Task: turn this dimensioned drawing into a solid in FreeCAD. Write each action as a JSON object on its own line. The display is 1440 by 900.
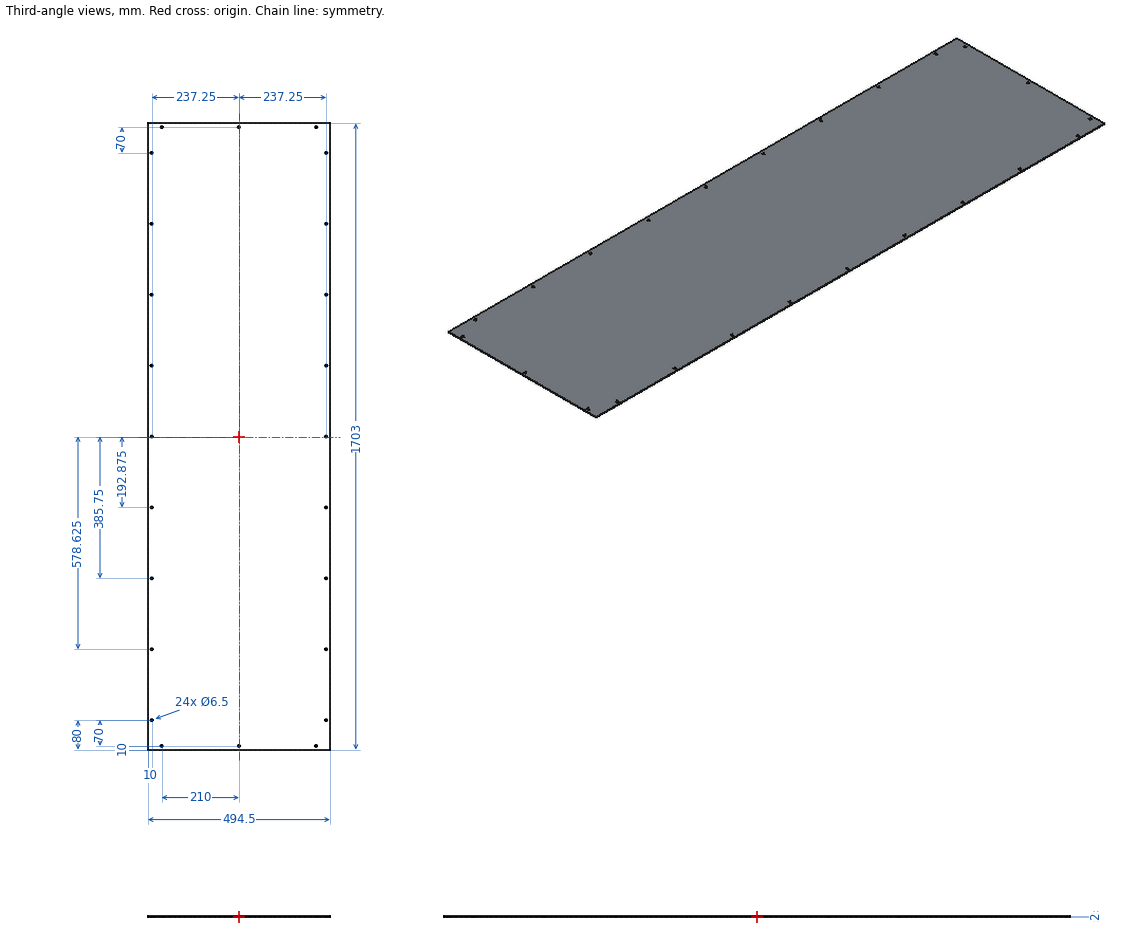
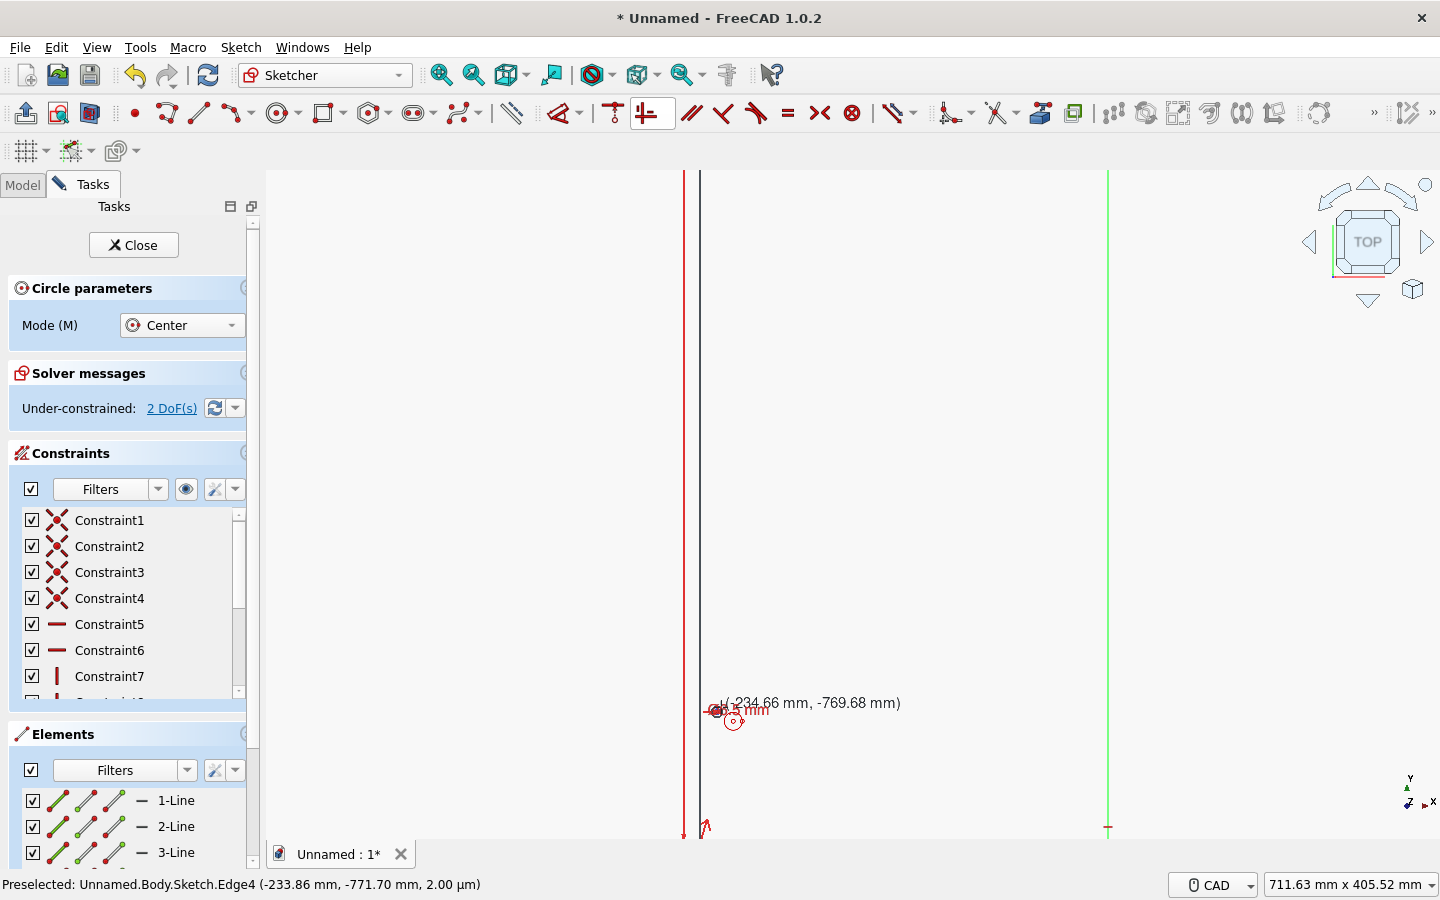
{"action": "scroll", "coordinate": [720, 716], "scroll_direction": "down", "scroll_amount": 9}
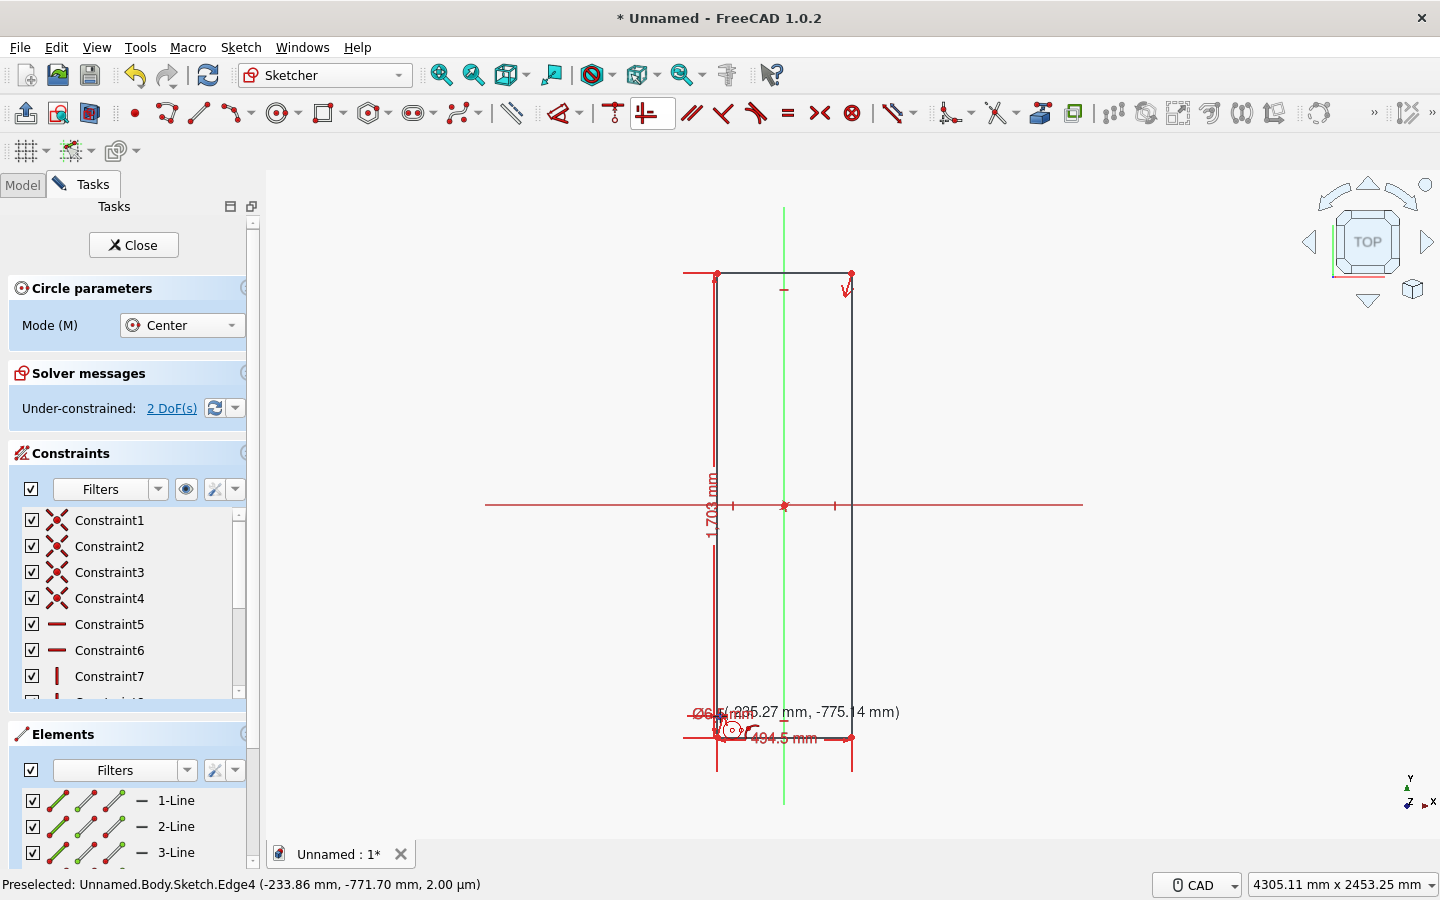
{"action": "scroll", "coordinate": [727, 735], "scroll_direction": "up", "scroll_amount": 17}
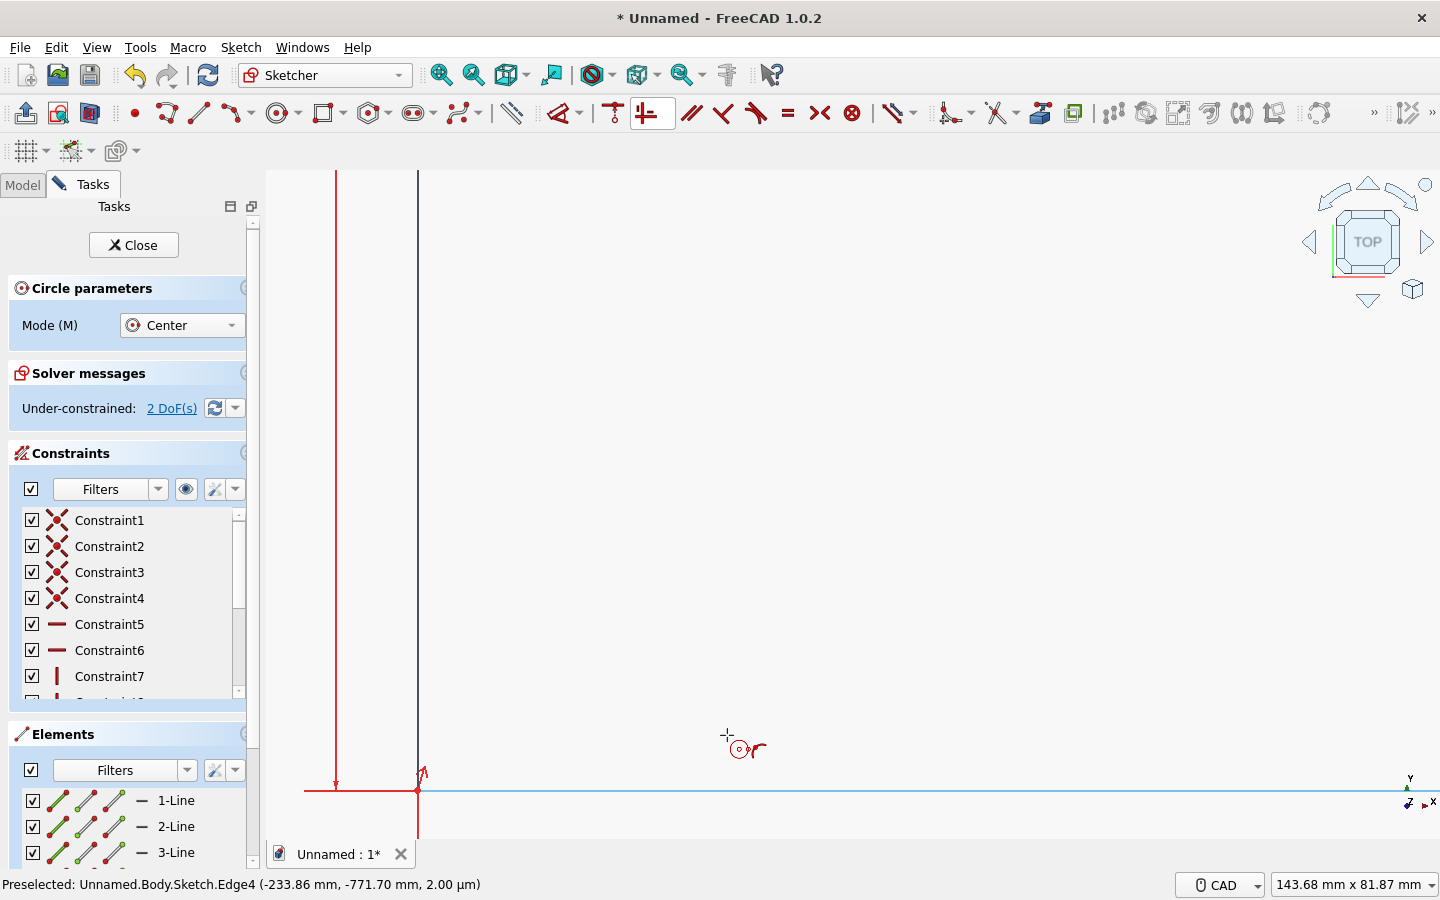
{"action": "scroll", "coordinate": [727, 735], "scroll_direction": "down", "scroll_amount": 17}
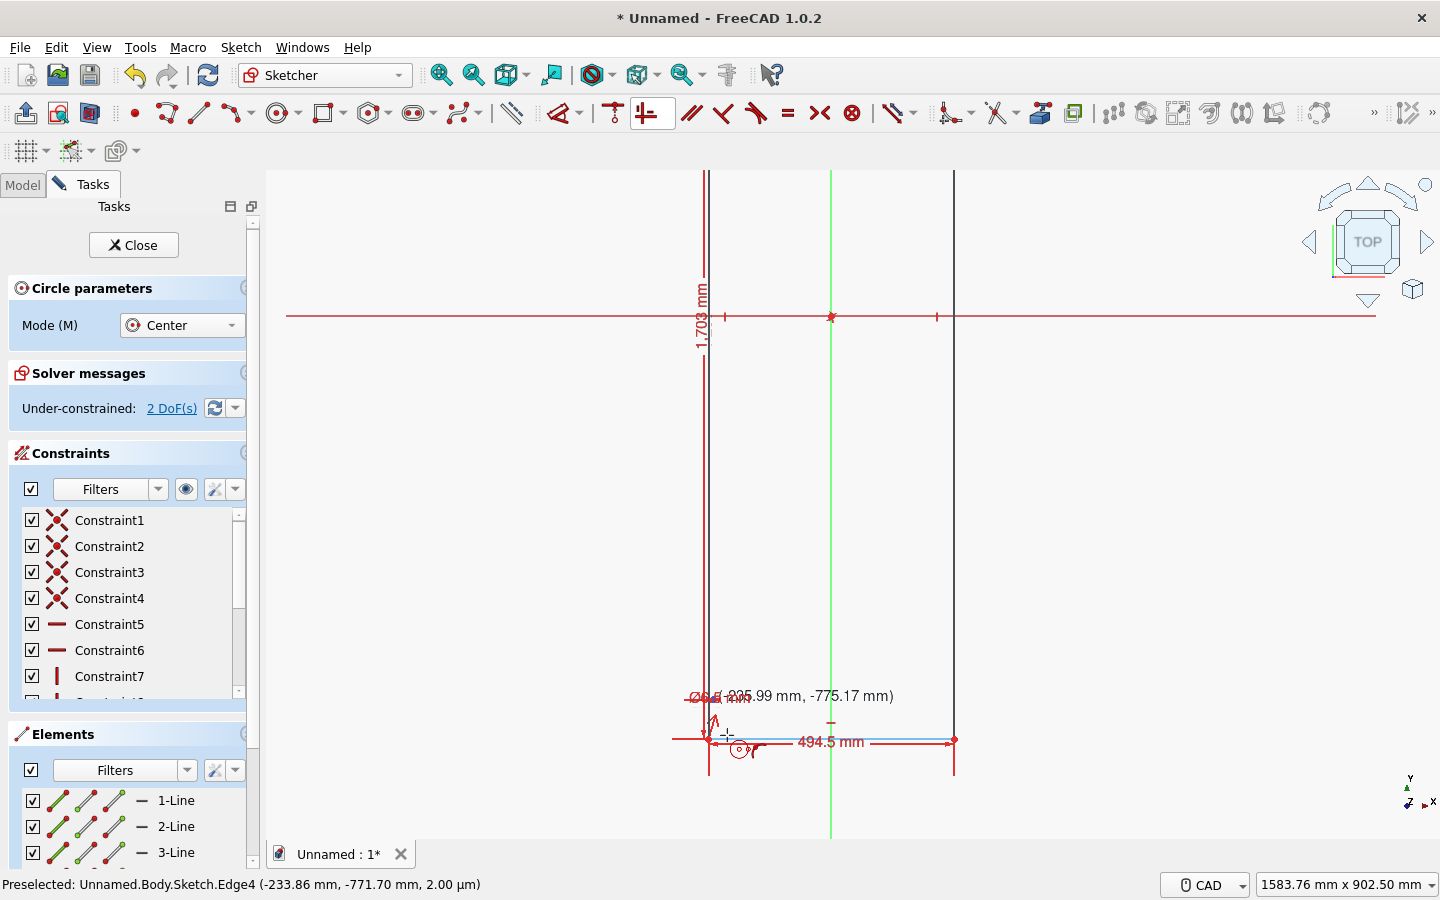
{"action": "scroll", "coordinate": [727, 735], "scroll_direction": "up", "scroll_amount": 9}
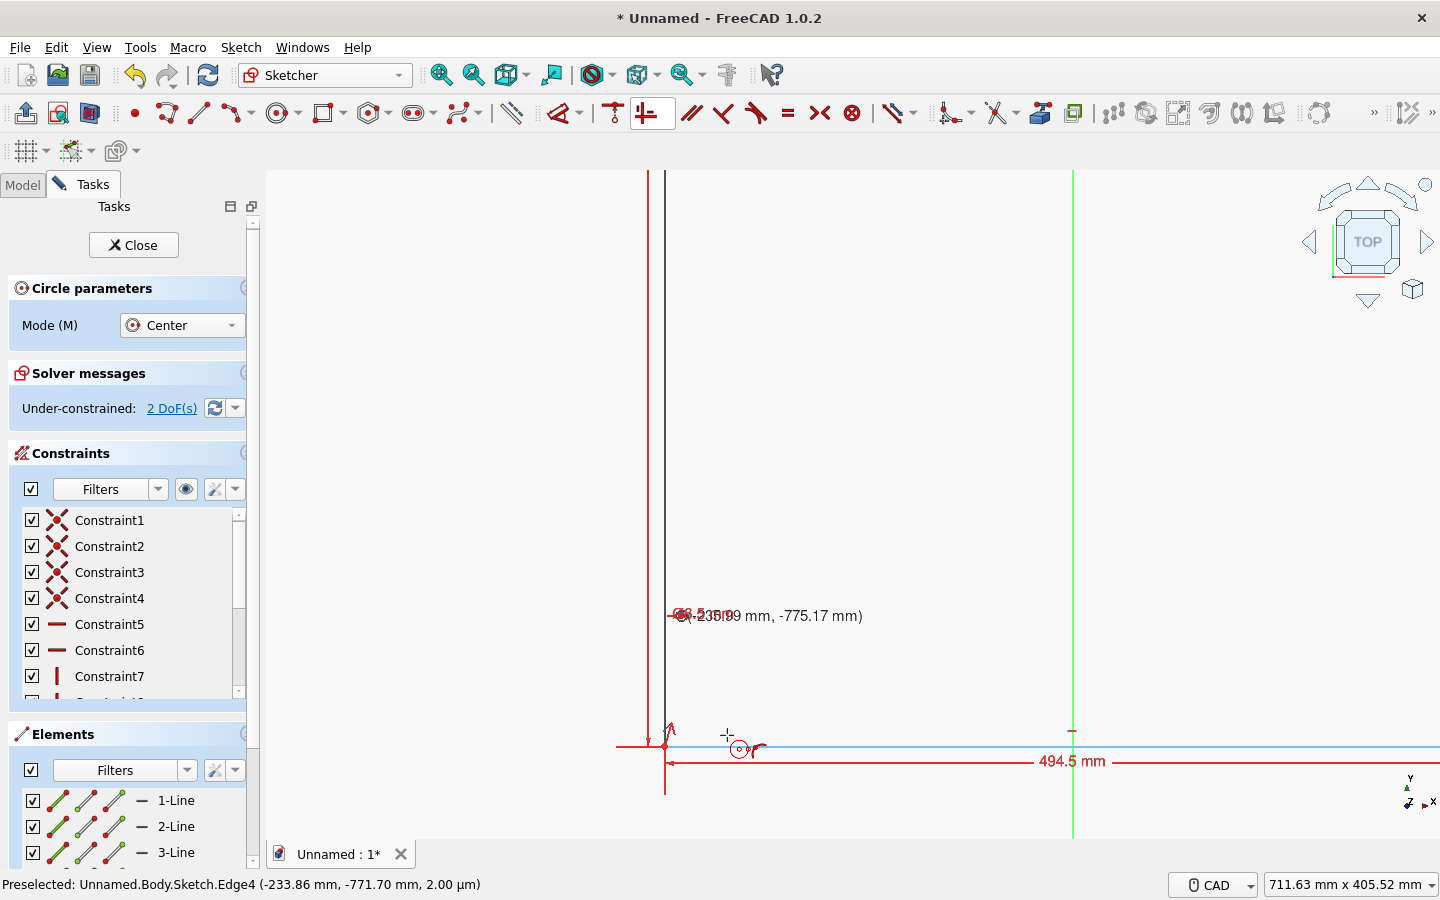
{"action": "left_click", "coordinate": [726, 730]}
{"action": "mouse_move", "coordinate": [730, 727]}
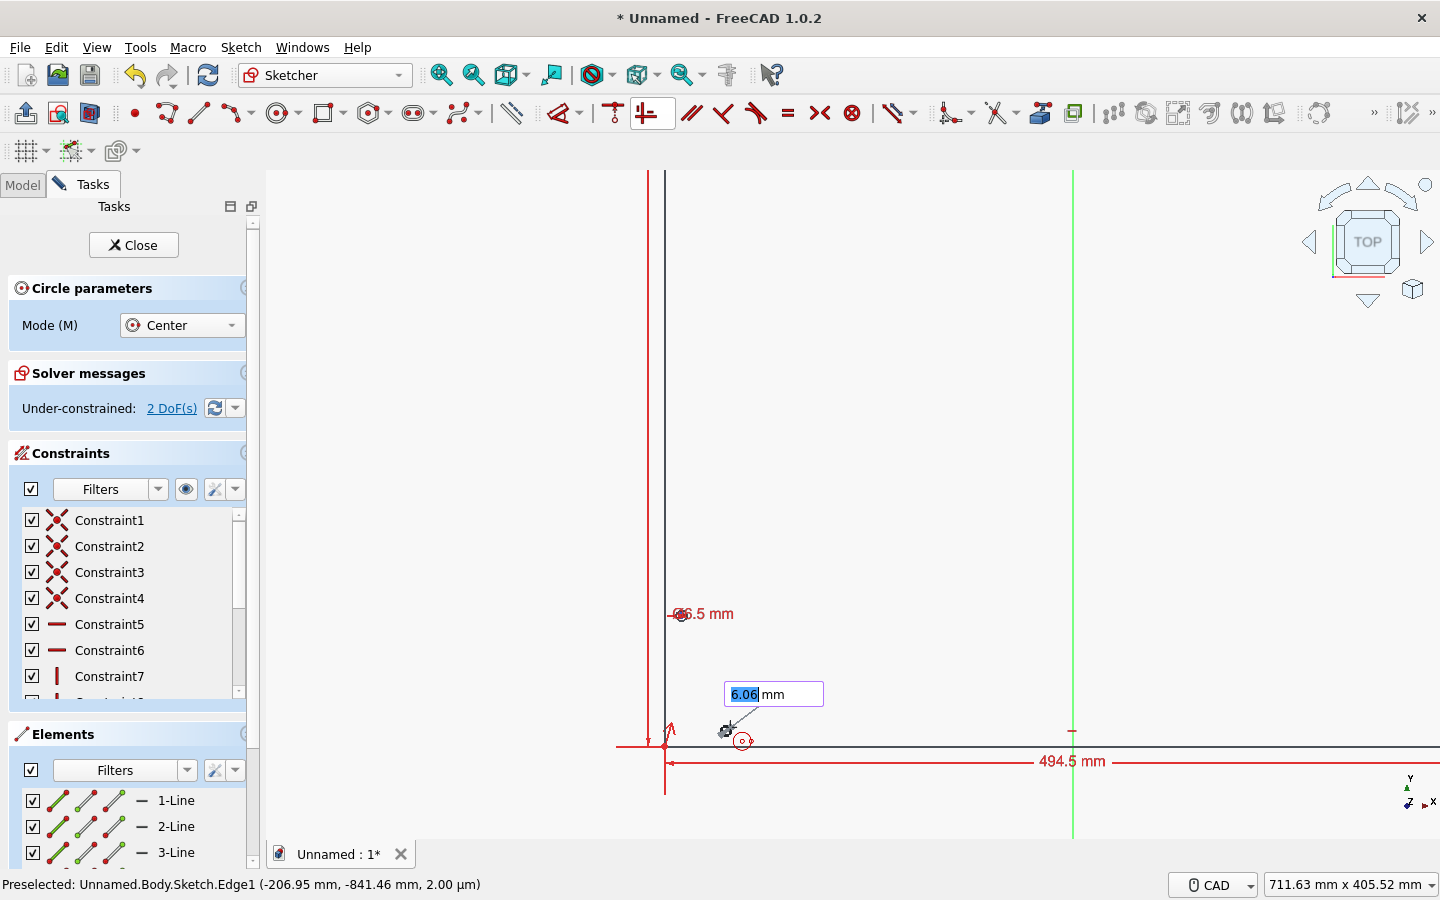
{"action": "type", "text": "6.5"}
{"action": "key", "text": "Return"}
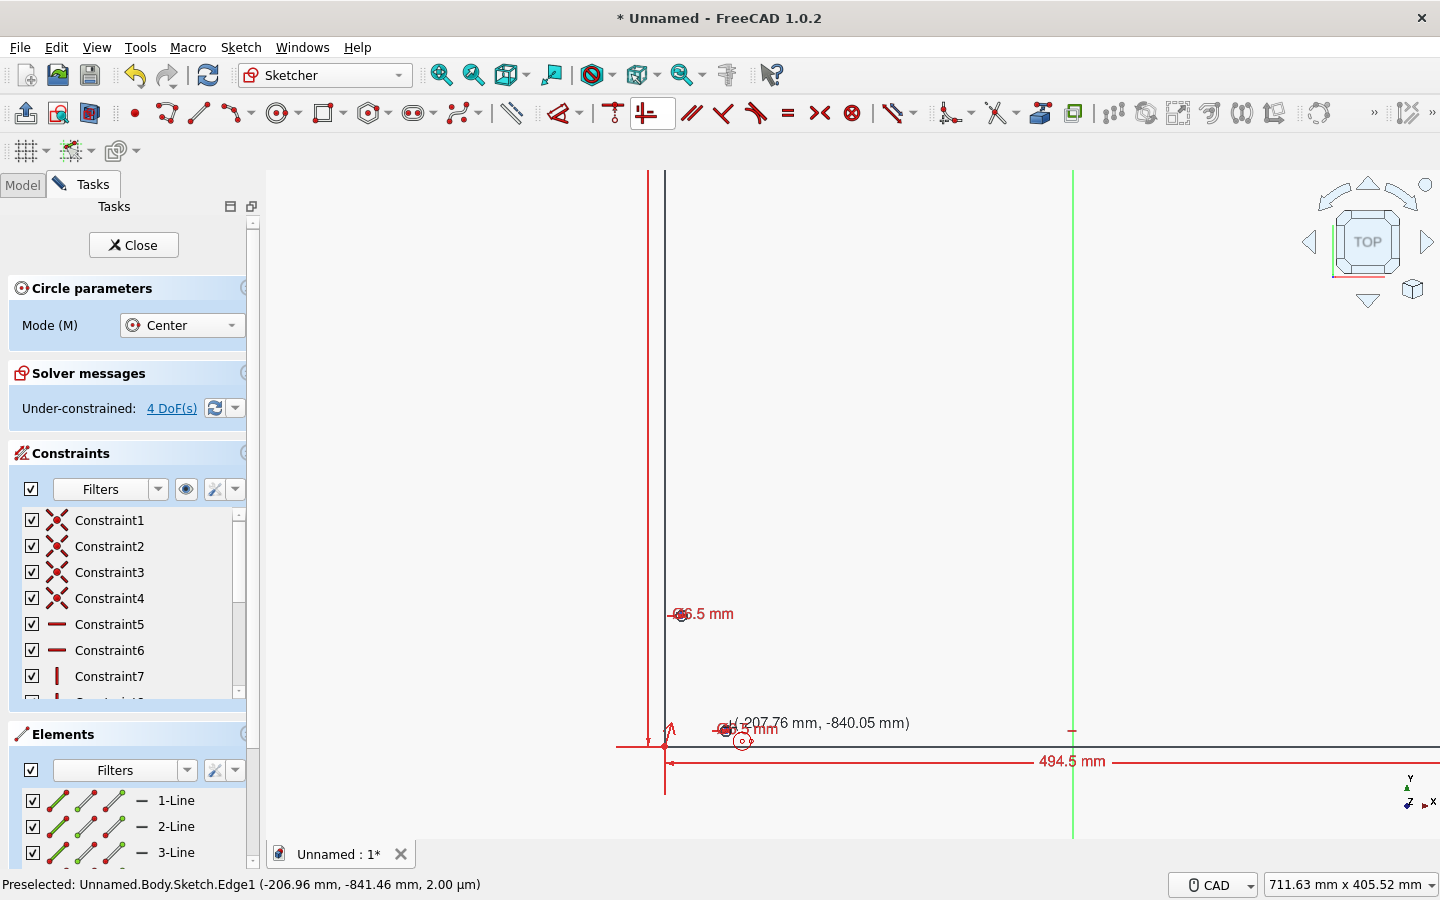
{"action": "scroll", "coordinate": [681, 297], "scroll_direction": "up", "scroll_amount": 8}